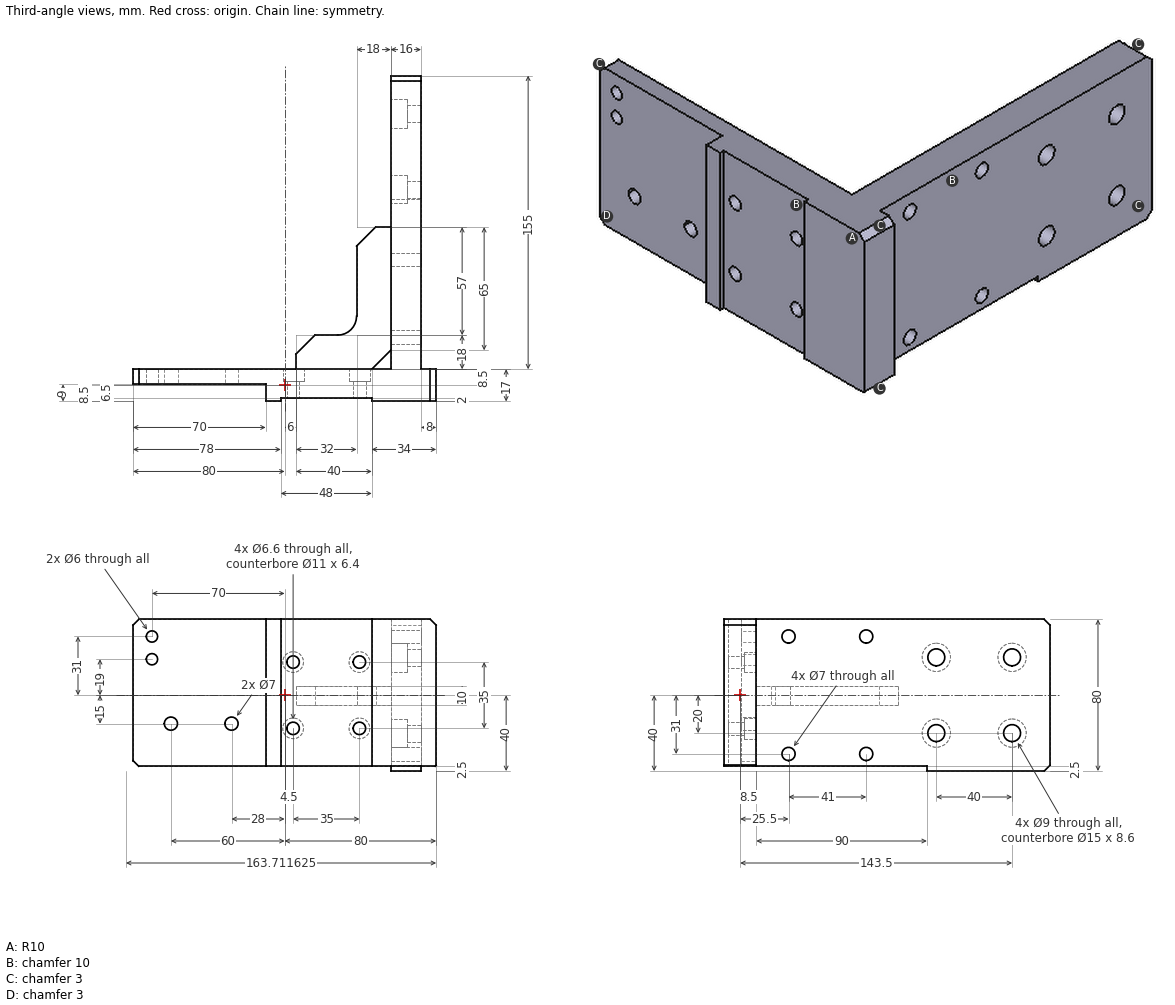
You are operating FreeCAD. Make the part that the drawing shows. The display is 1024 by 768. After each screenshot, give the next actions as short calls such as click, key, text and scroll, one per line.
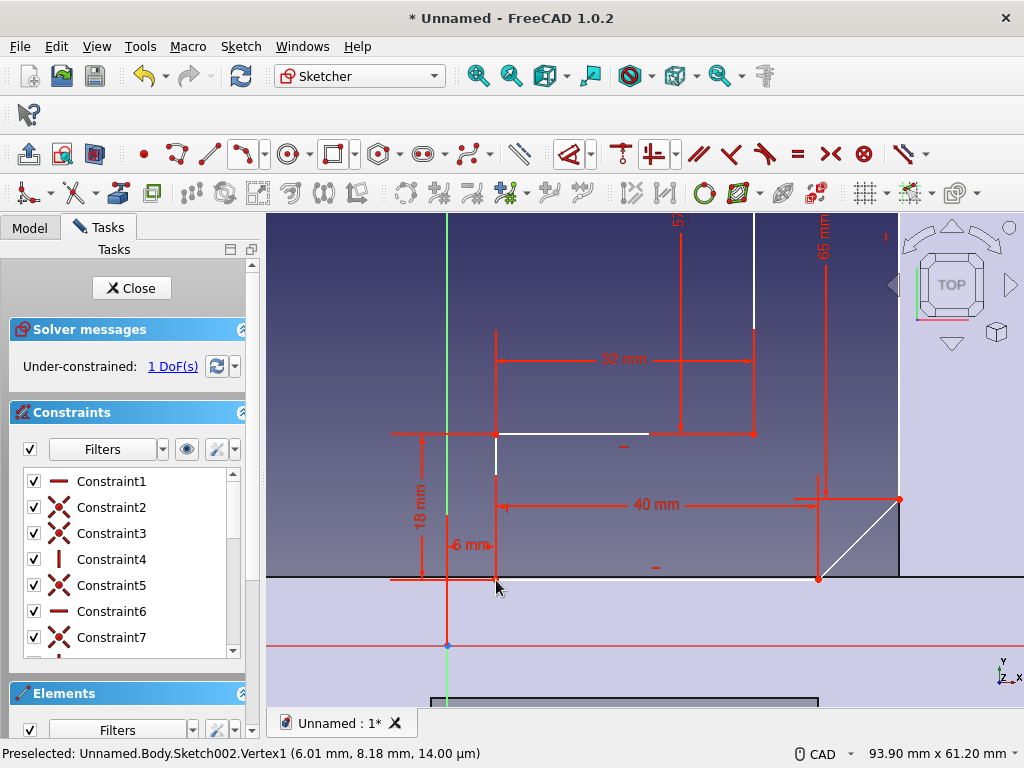
click(496, 580)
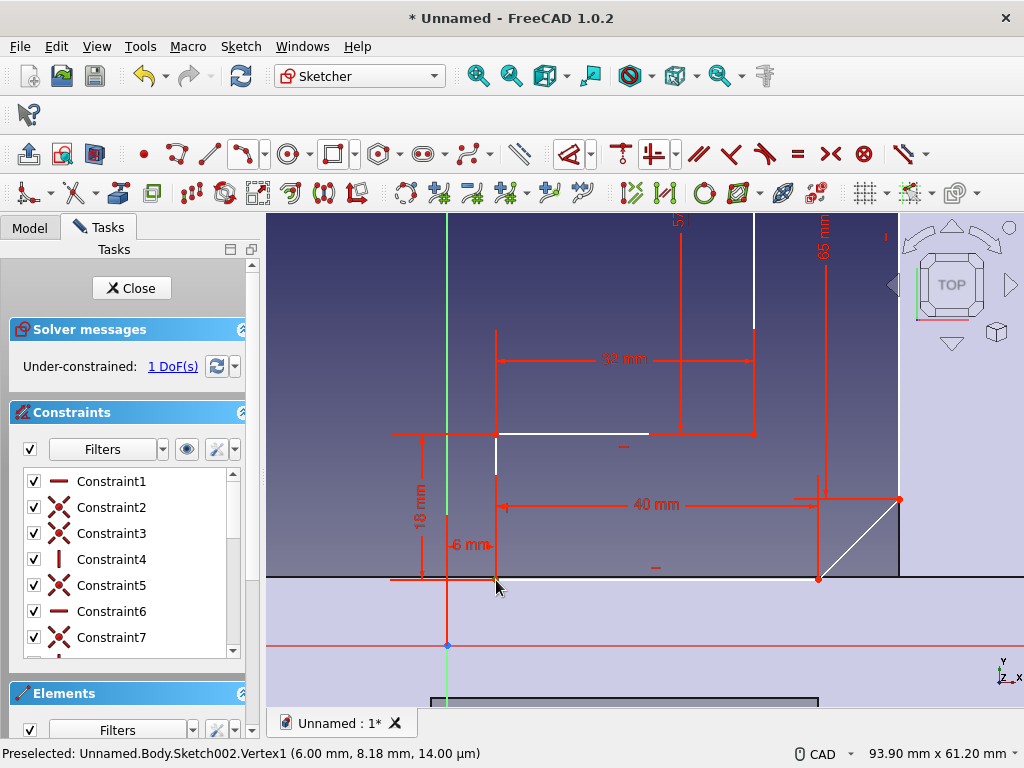
key(i)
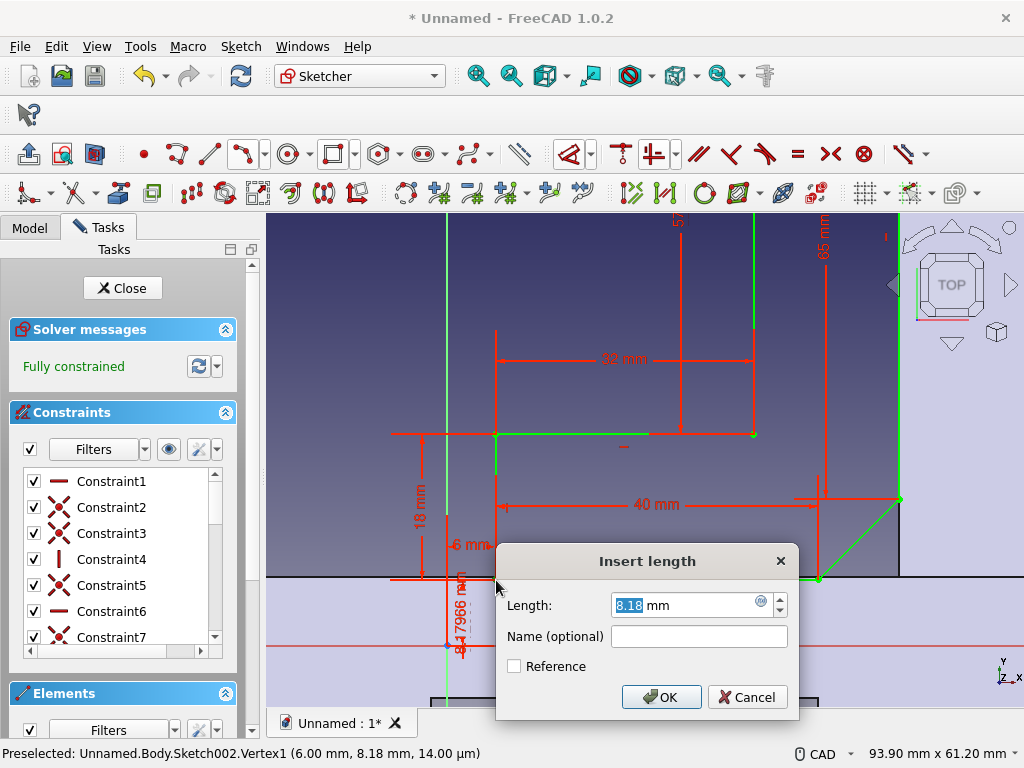
text(8.5)
key(Return)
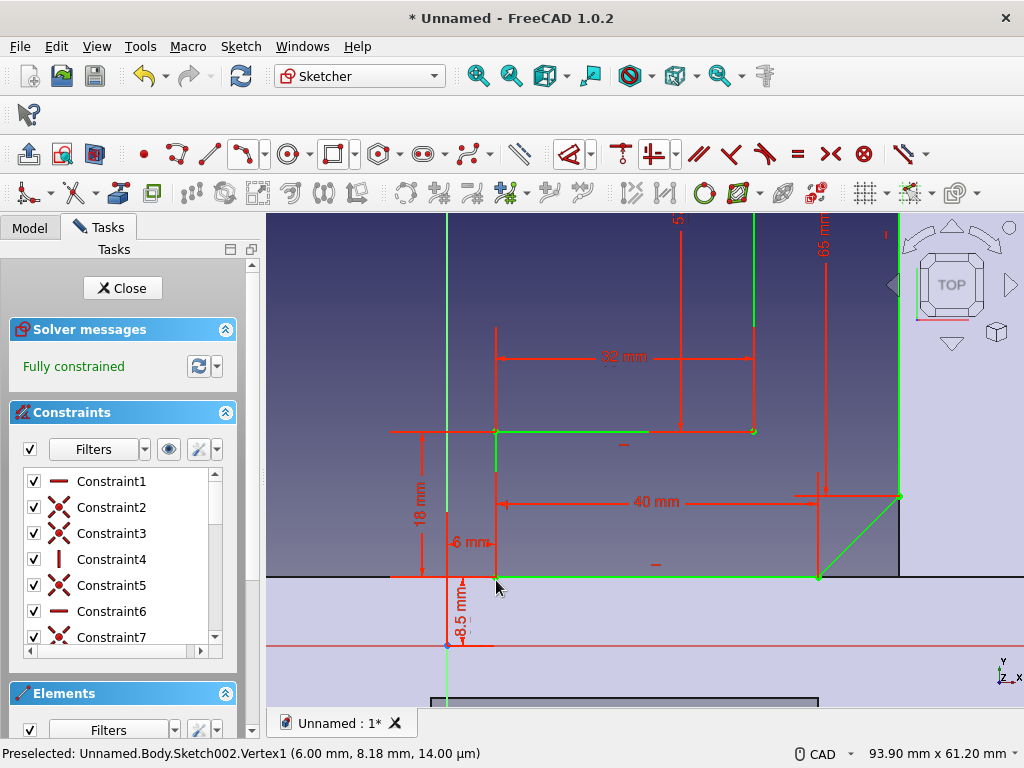
click(123, 288)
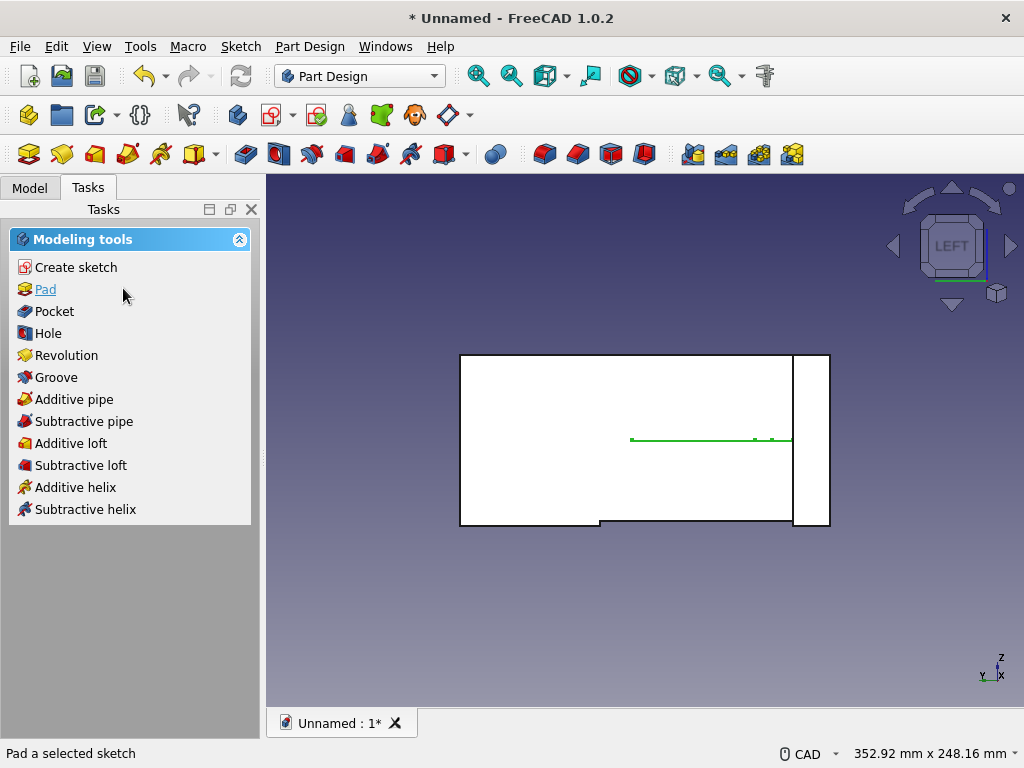
click(29, 154)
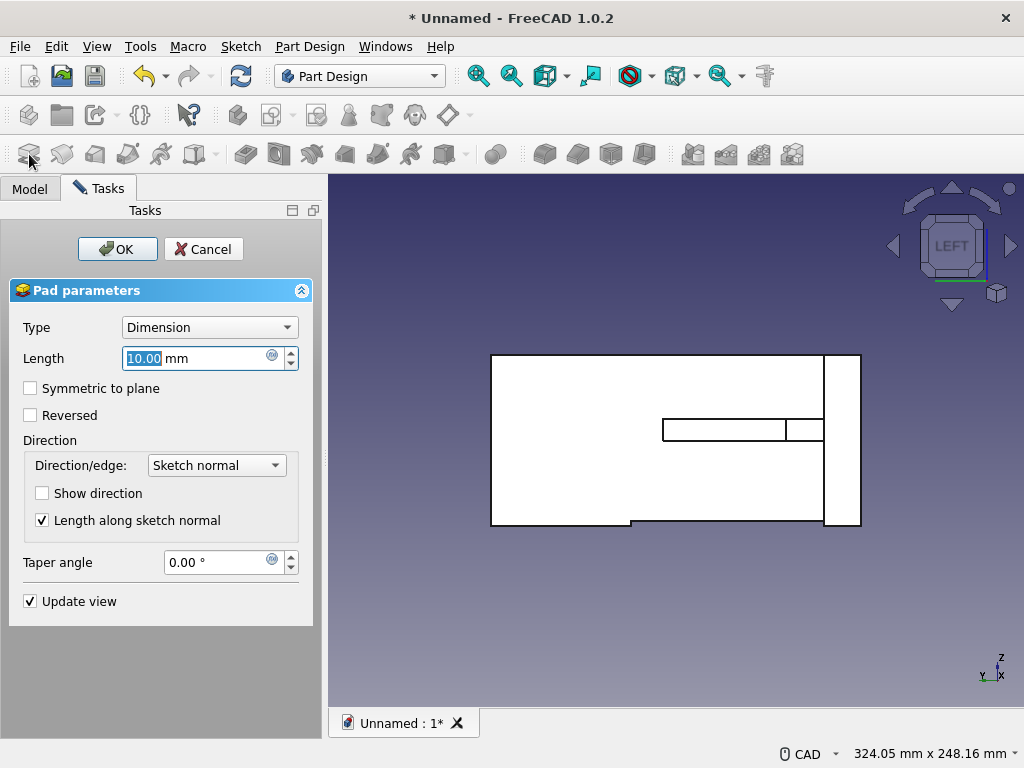
text(10)
key(Tab)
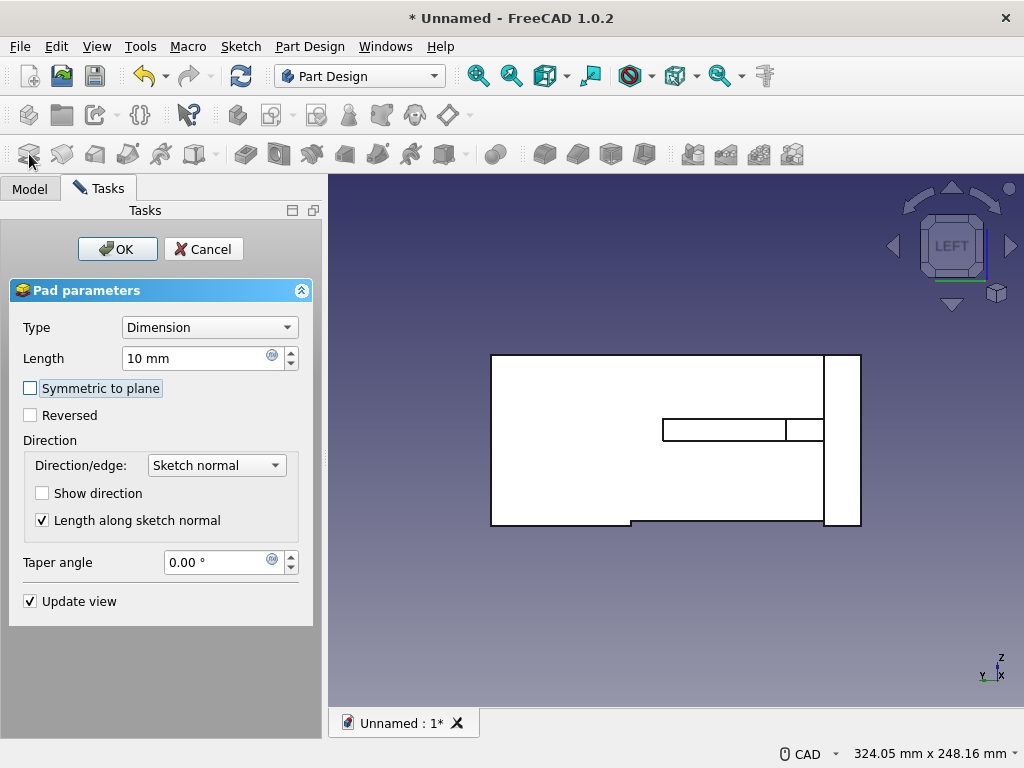
click(31, 388)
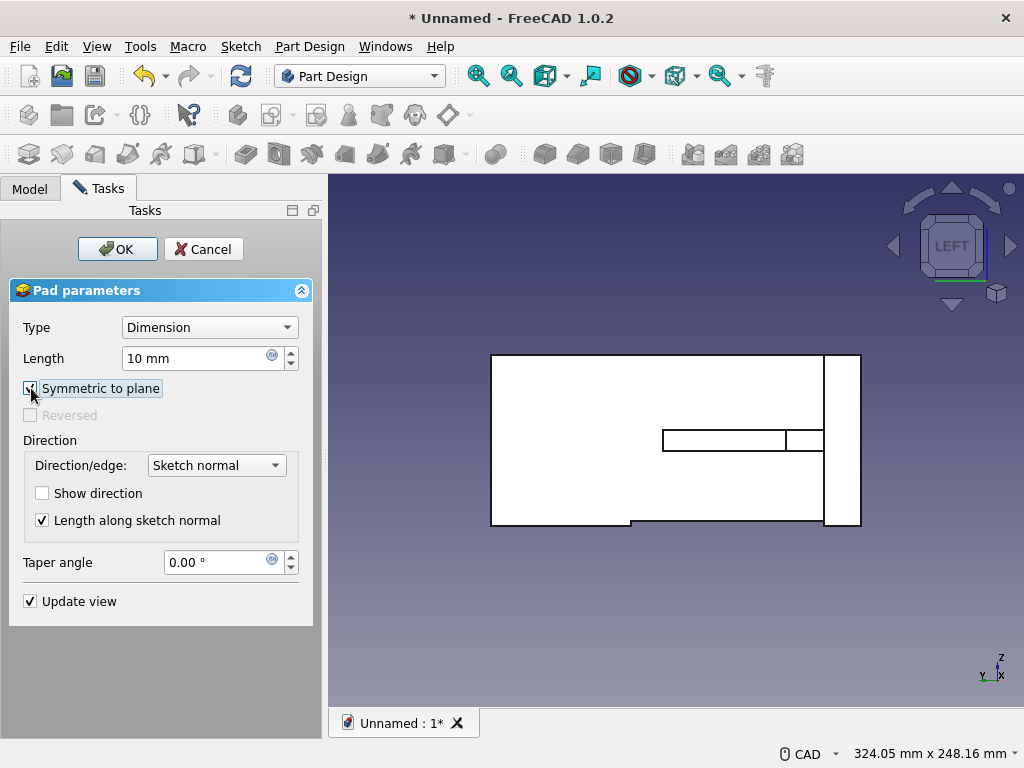
click(118, 249)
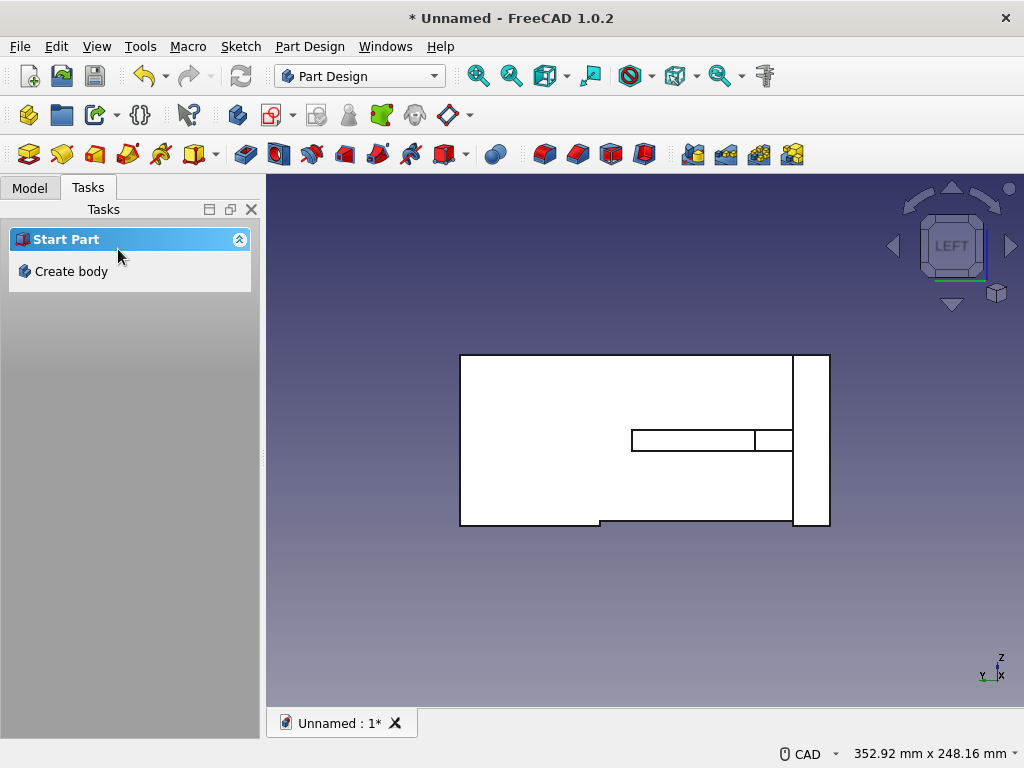
scroll(755, 439, up, 4)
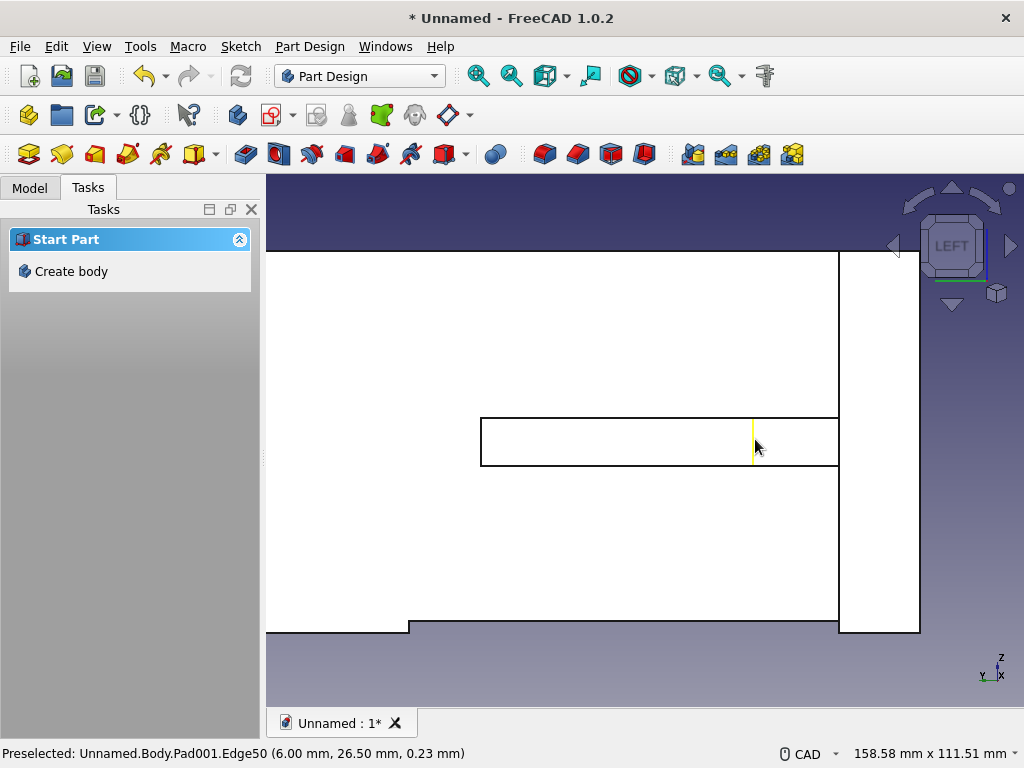
key(v)
key(f)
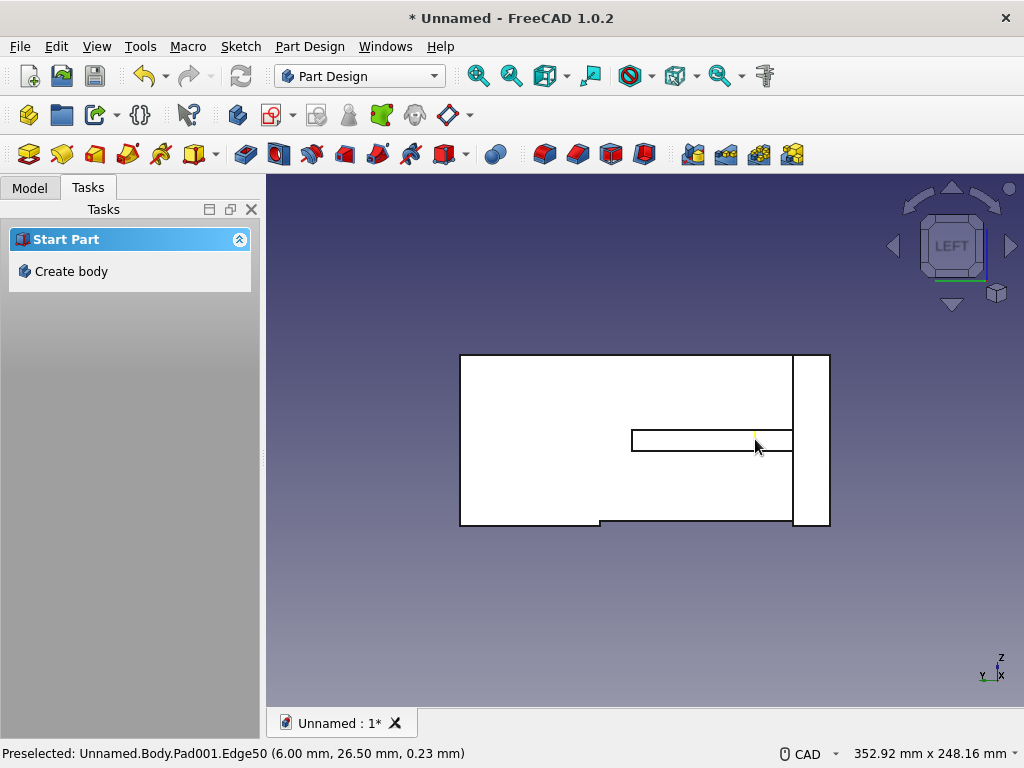
key(0)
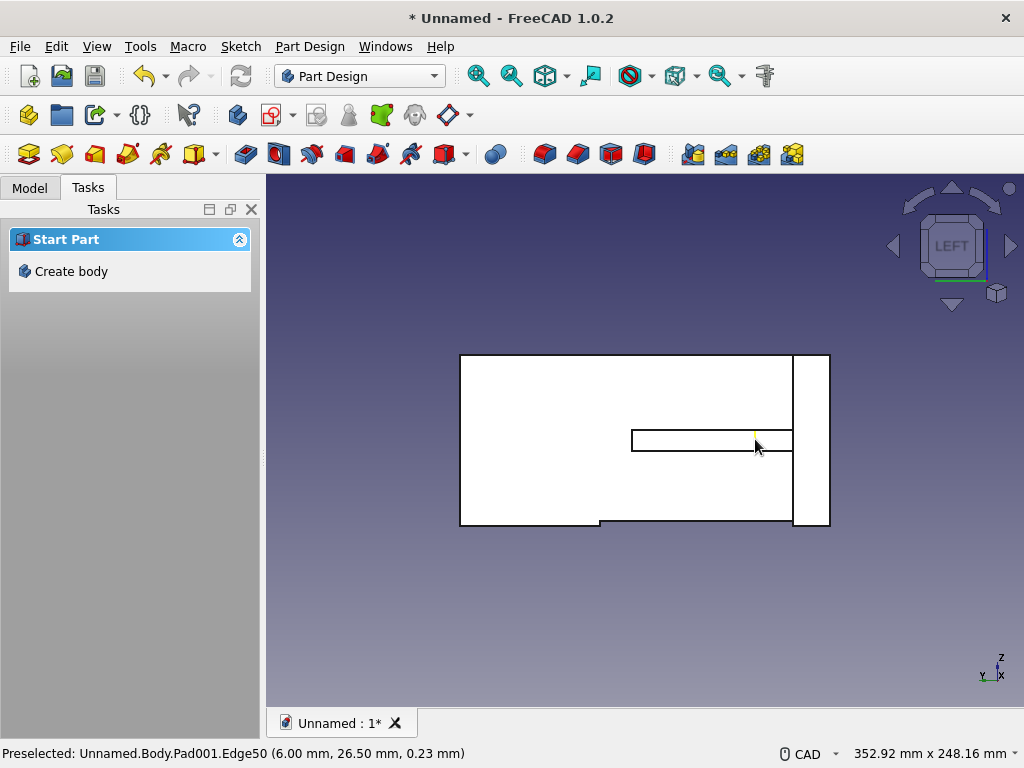
scroll(625, 518, up, 4)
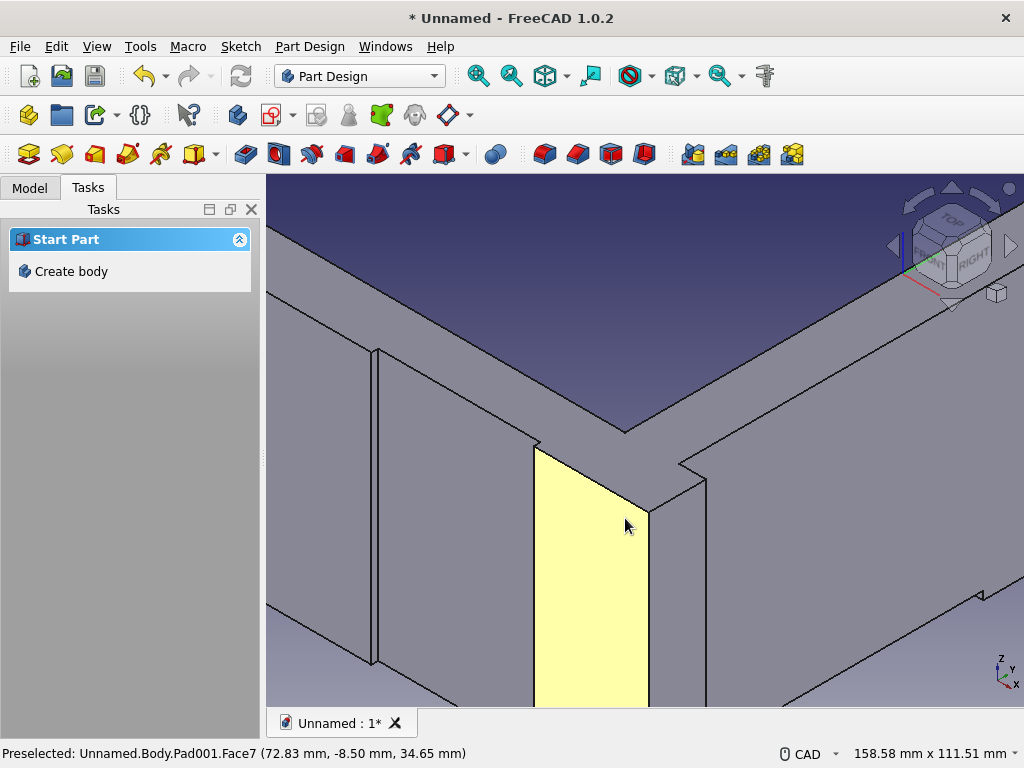
click(479, 76)